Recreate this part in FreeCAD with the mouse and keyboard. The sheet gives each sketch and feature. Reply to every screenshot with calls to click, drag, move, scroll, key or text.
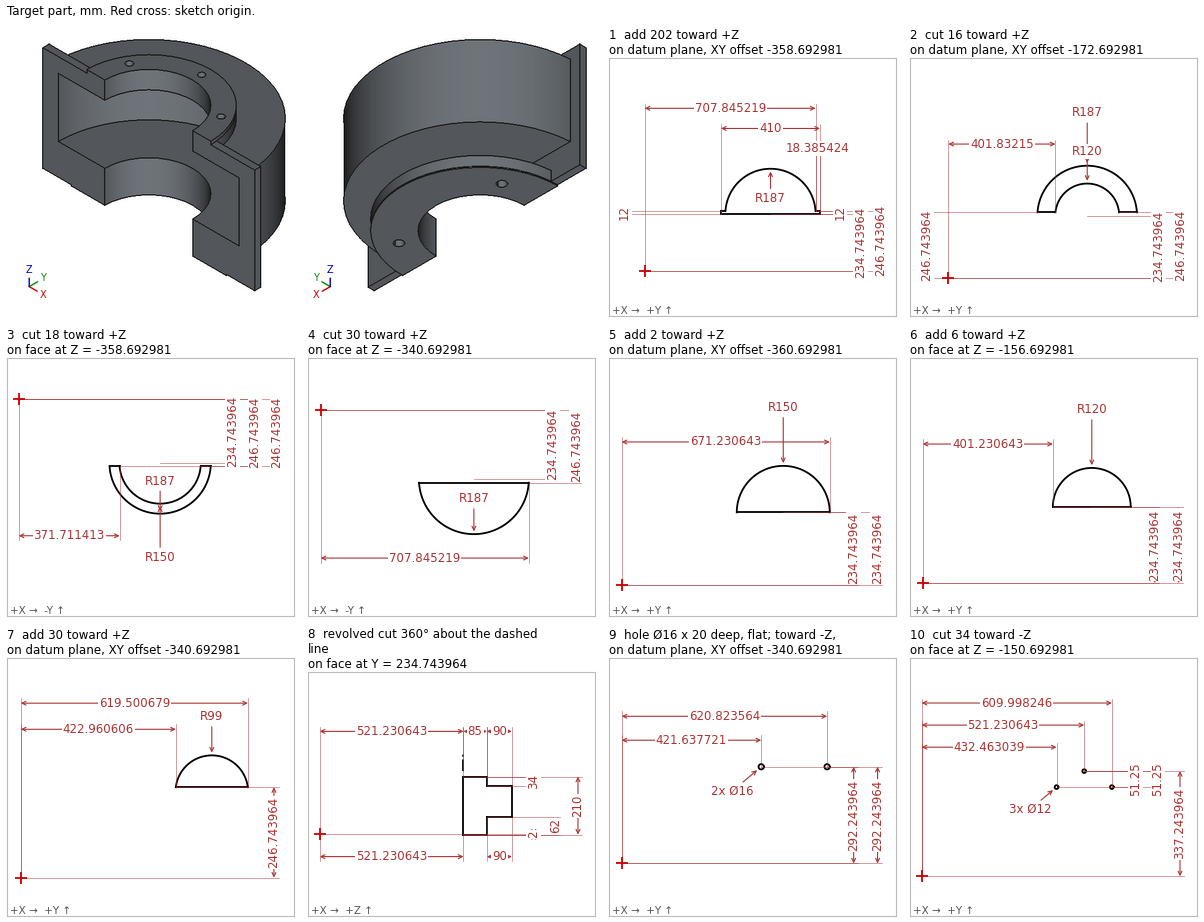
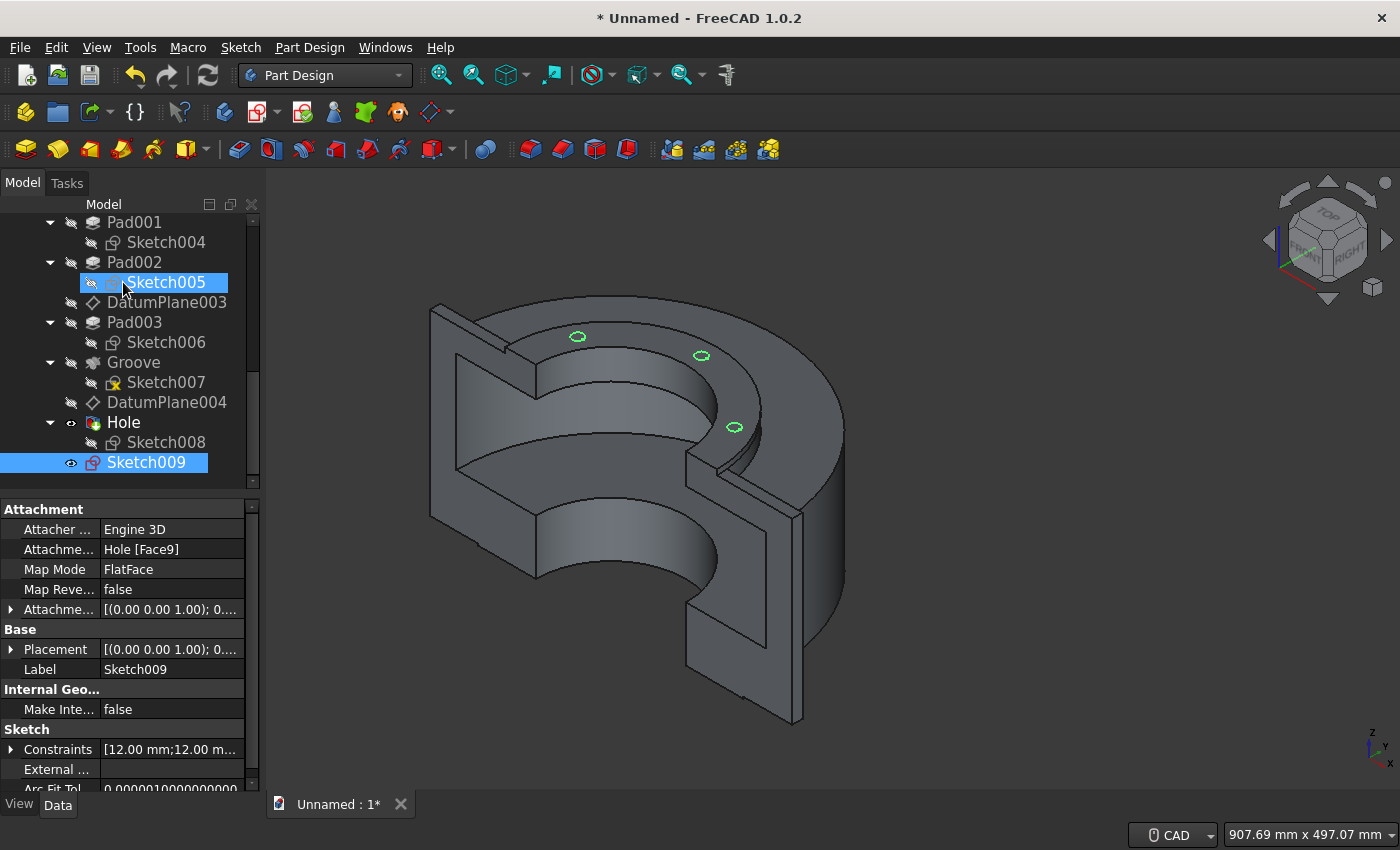
click(240, 150)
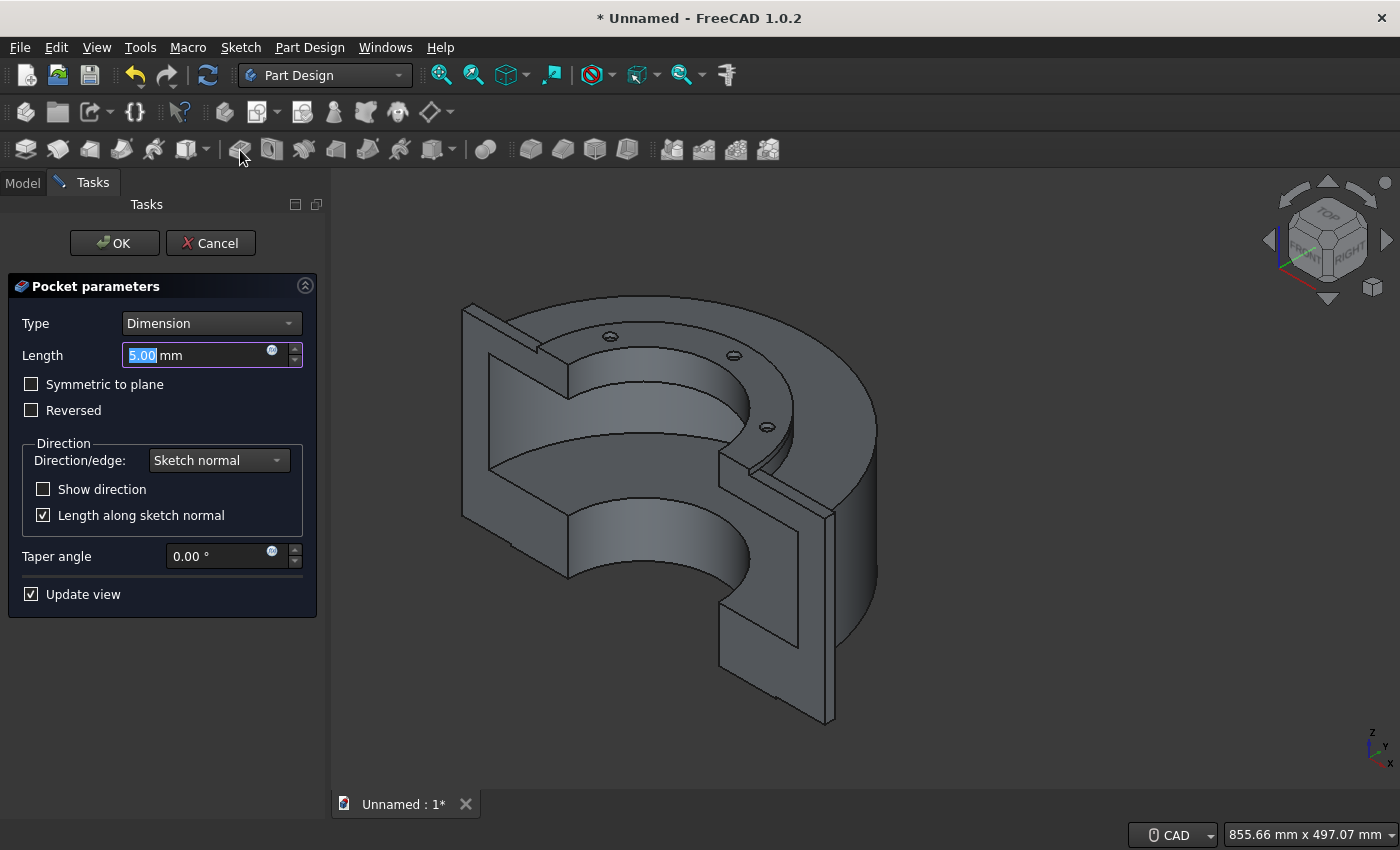
text(34)
key(Tab)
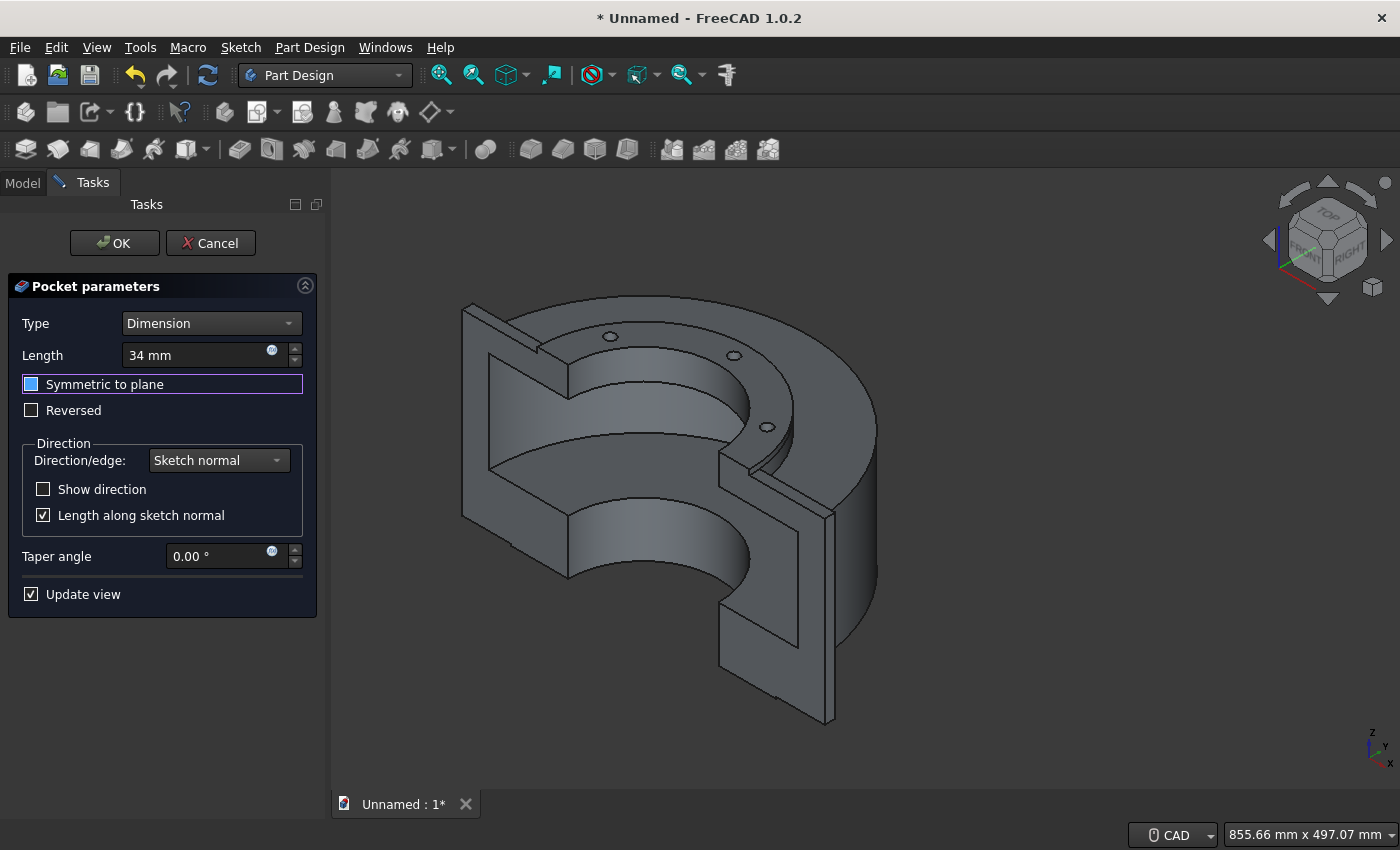
click(115, 243)